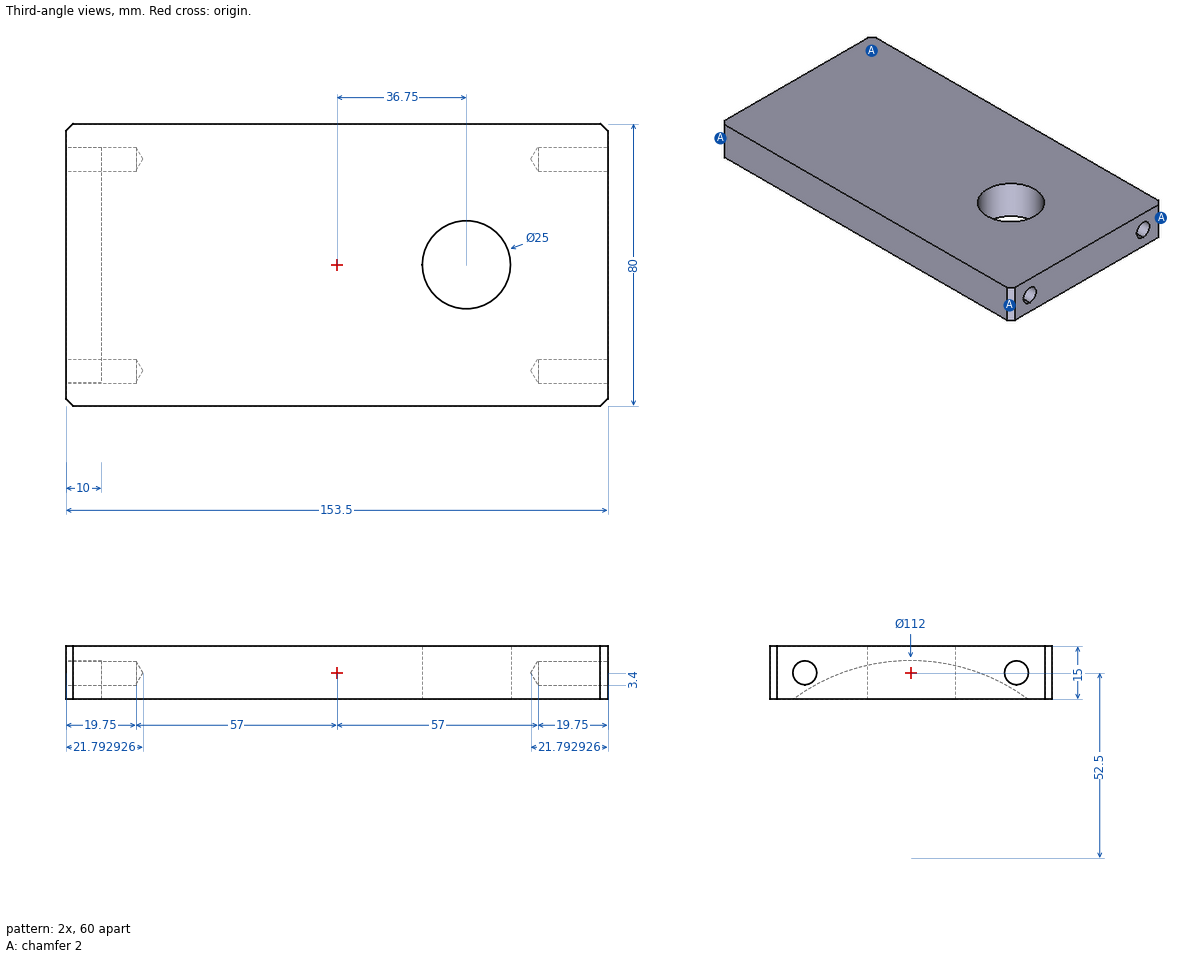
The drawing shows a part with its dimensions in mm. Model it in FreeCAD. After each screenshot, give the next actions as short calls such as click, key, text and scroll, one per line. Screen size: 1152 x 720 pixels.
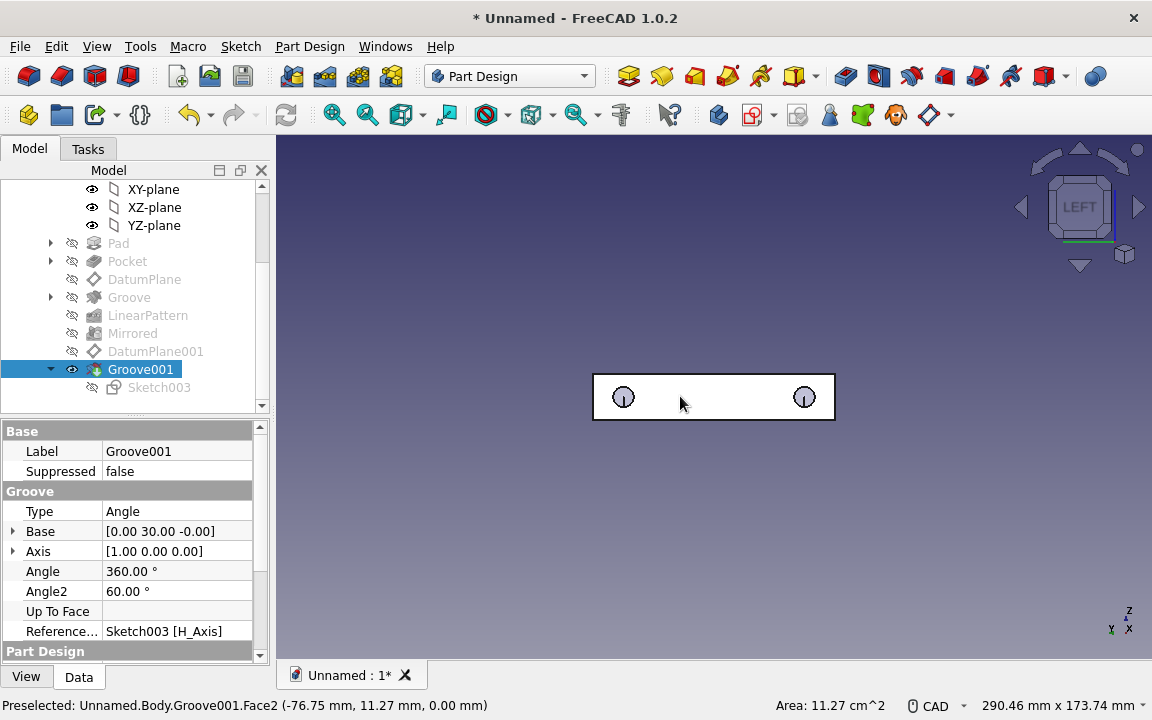
click(752, 116)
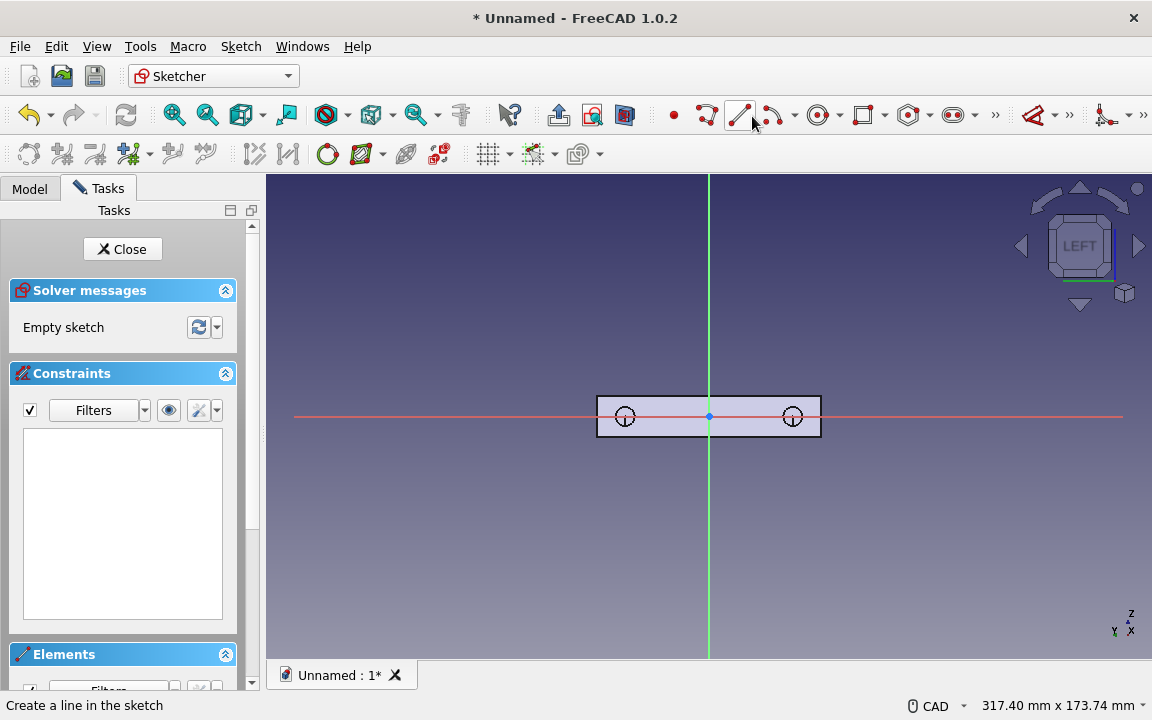
scroll(501, 202, down, 2)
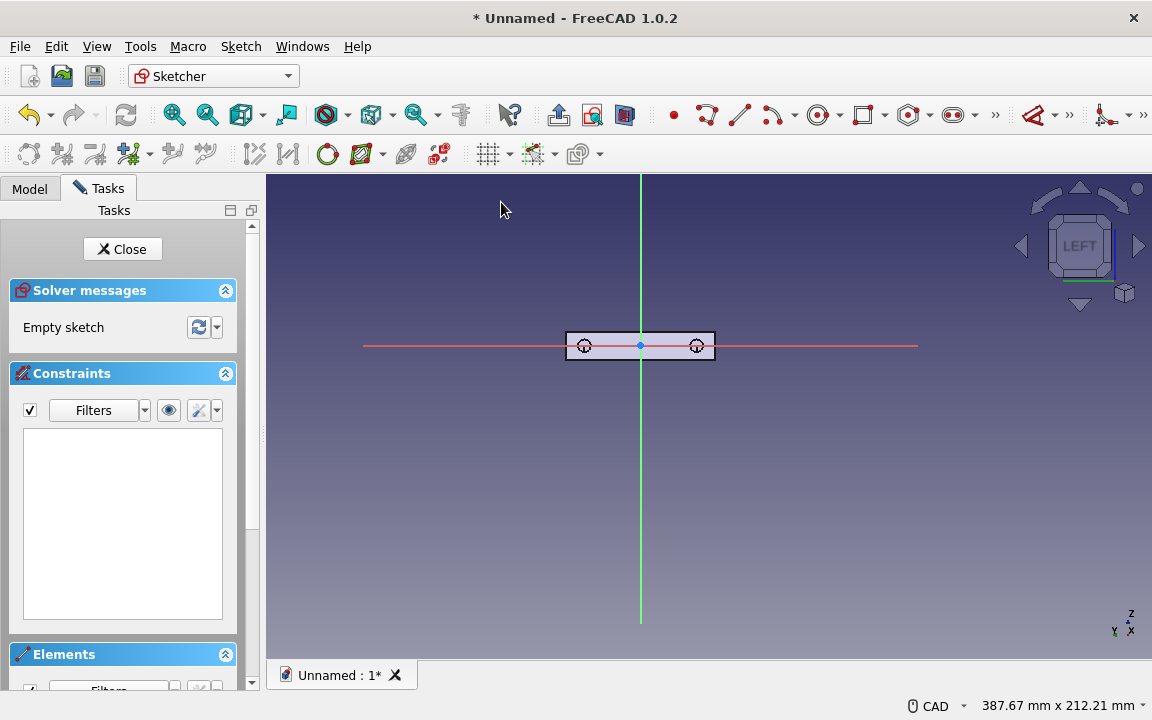
scroll(641, 500, up, 2)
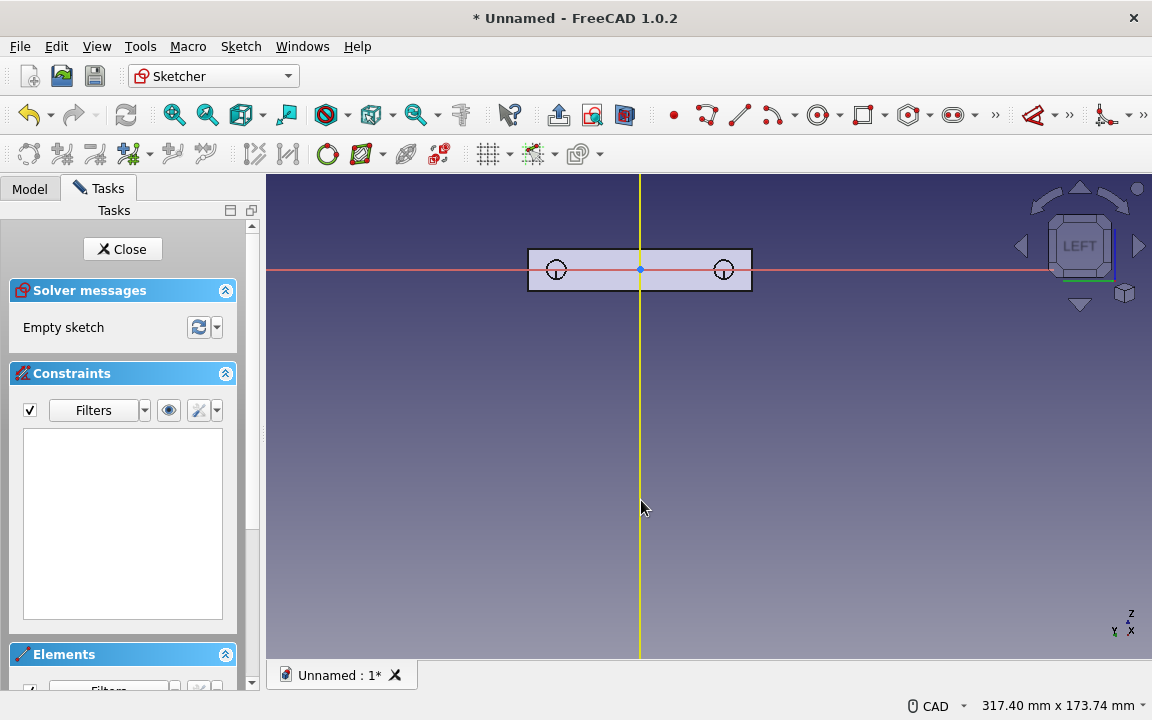
click(818, 116)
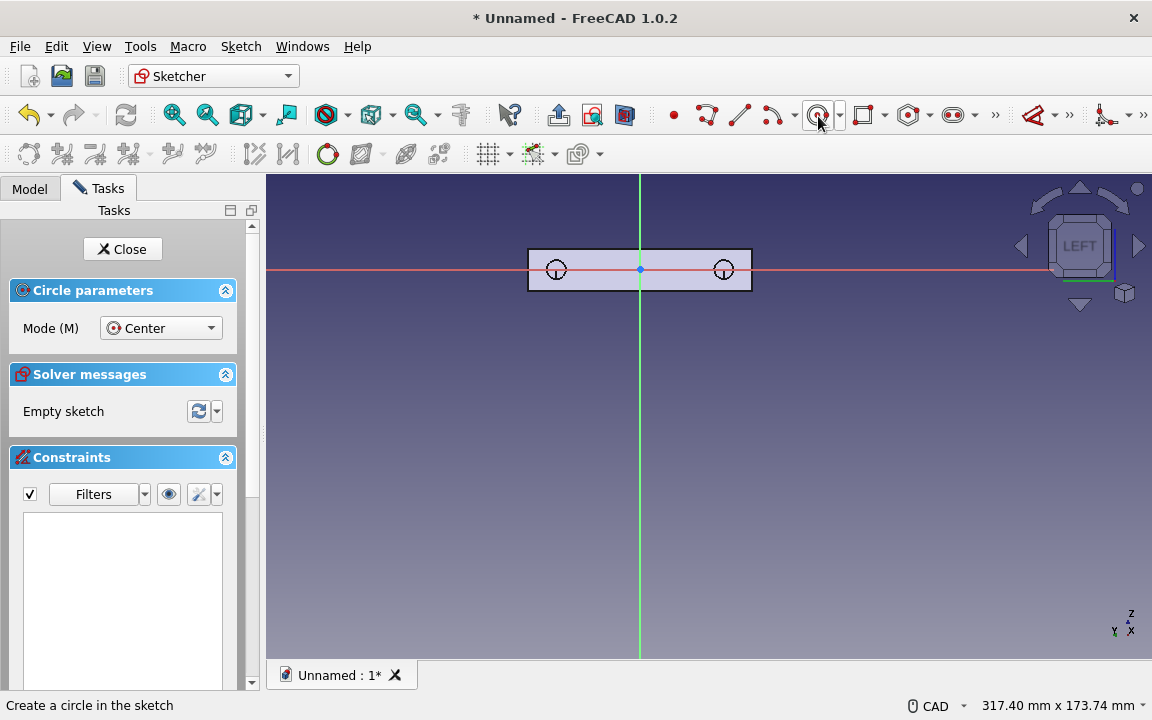
click(640, 416)
move(751, 306)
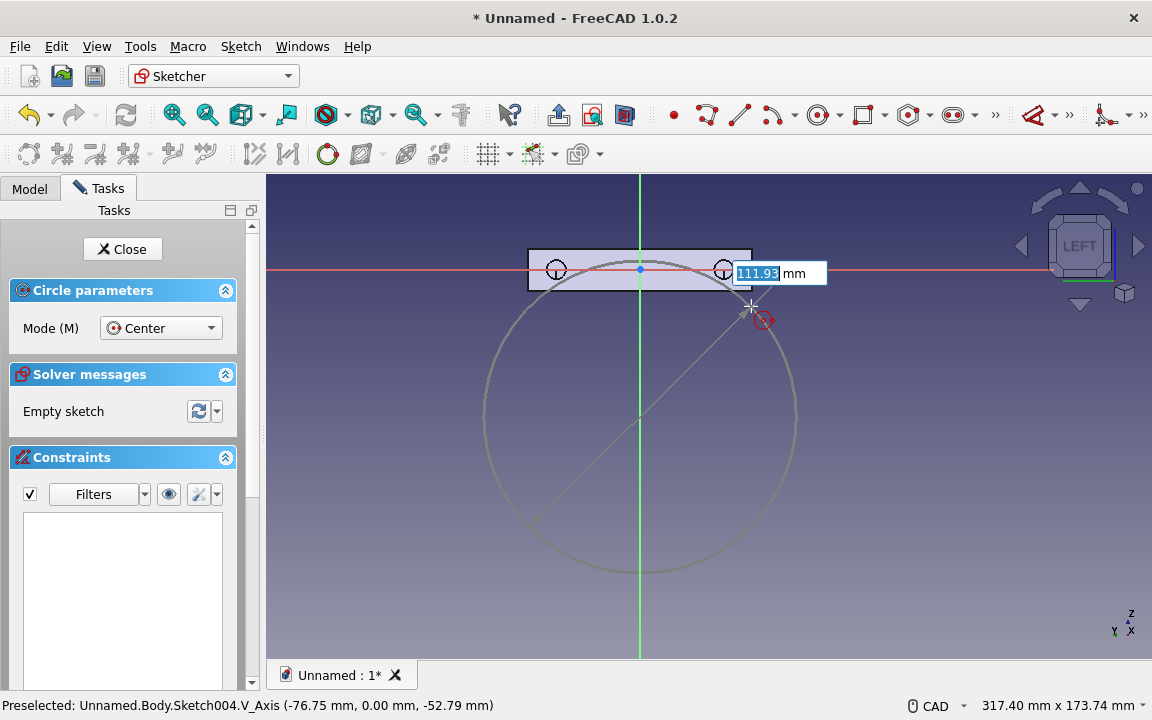
text(112)
key(Return)
key(Escape)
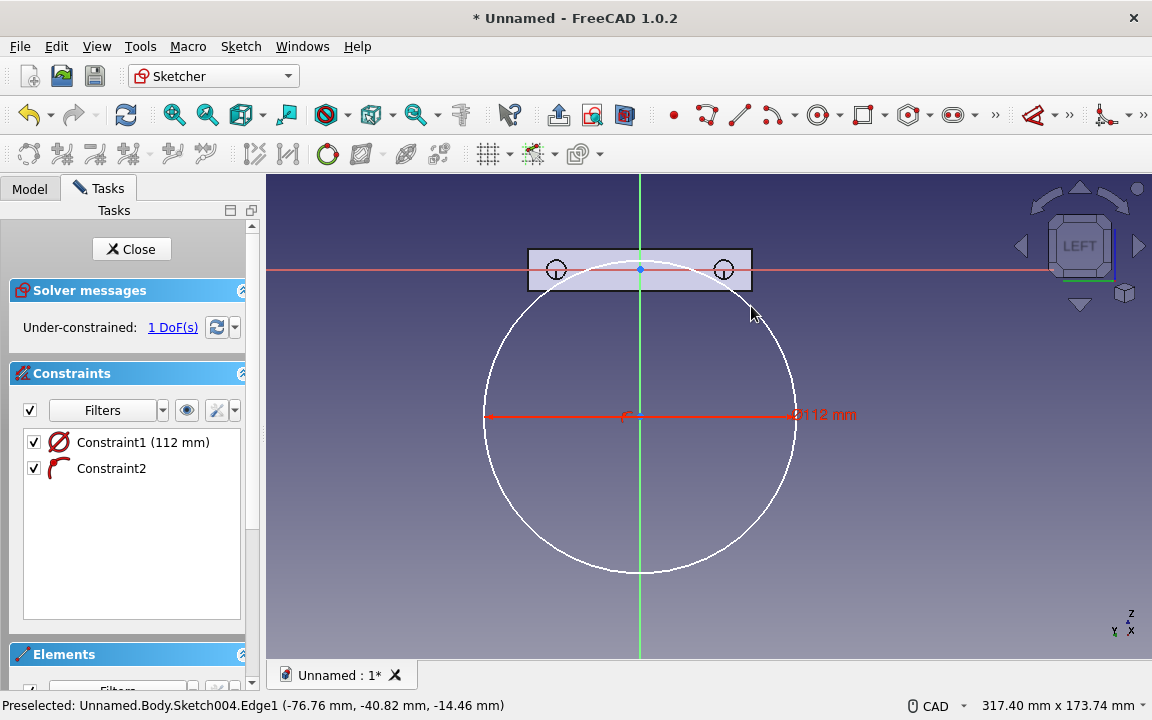
click(1032, 116)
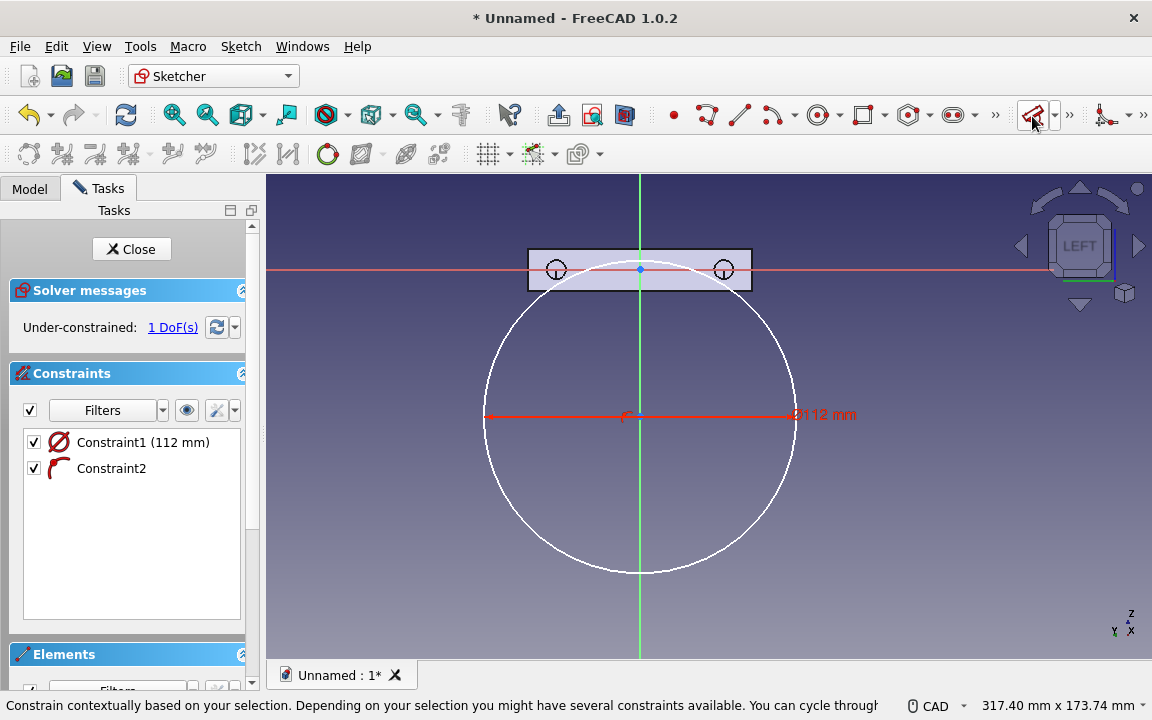
click(640, 417)
click(674, 343)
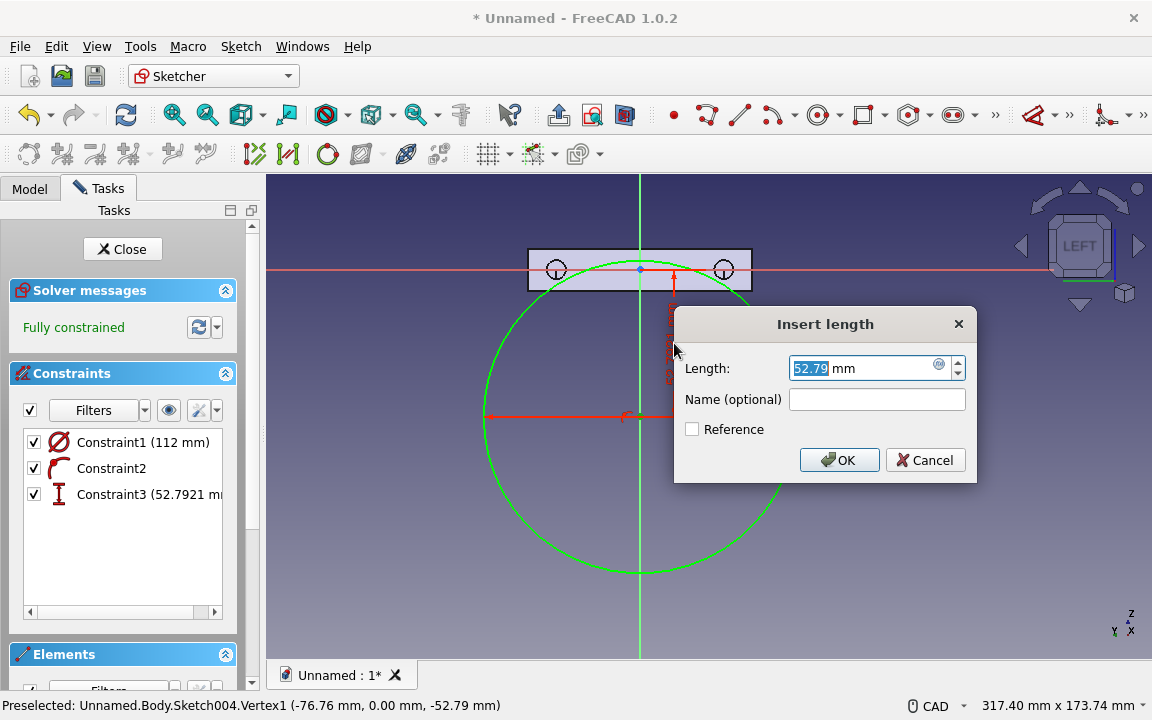
text(52.5)
key(Return)
key(Escape)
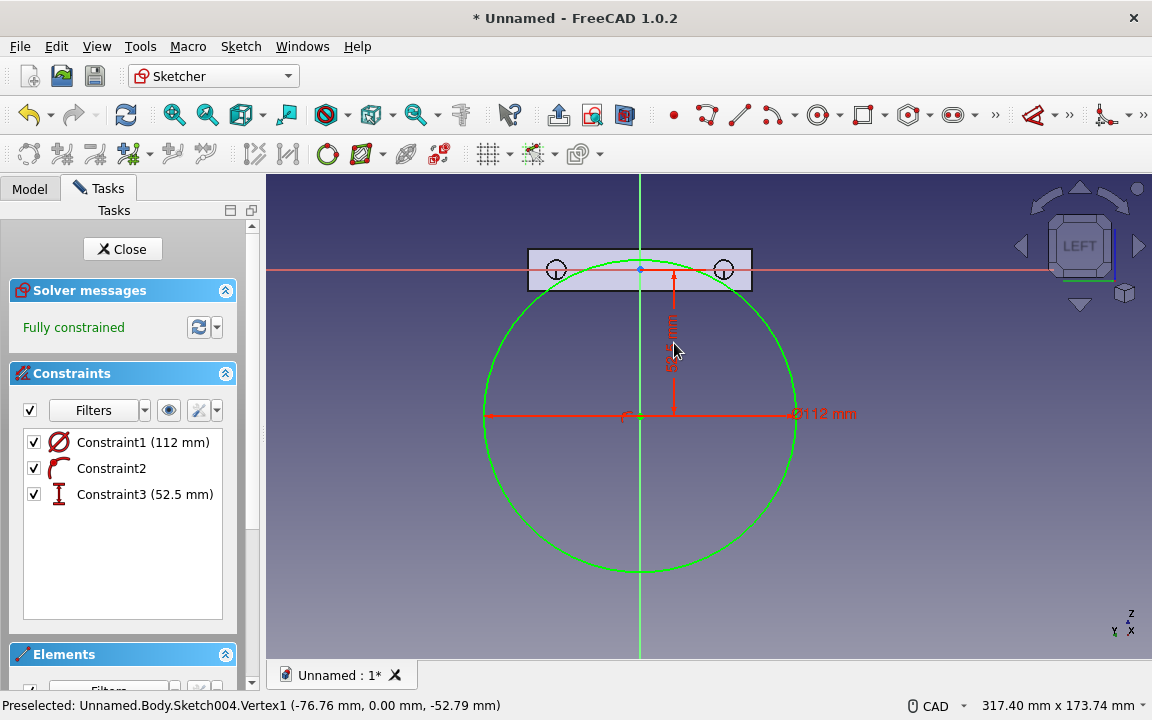
click(123, 249)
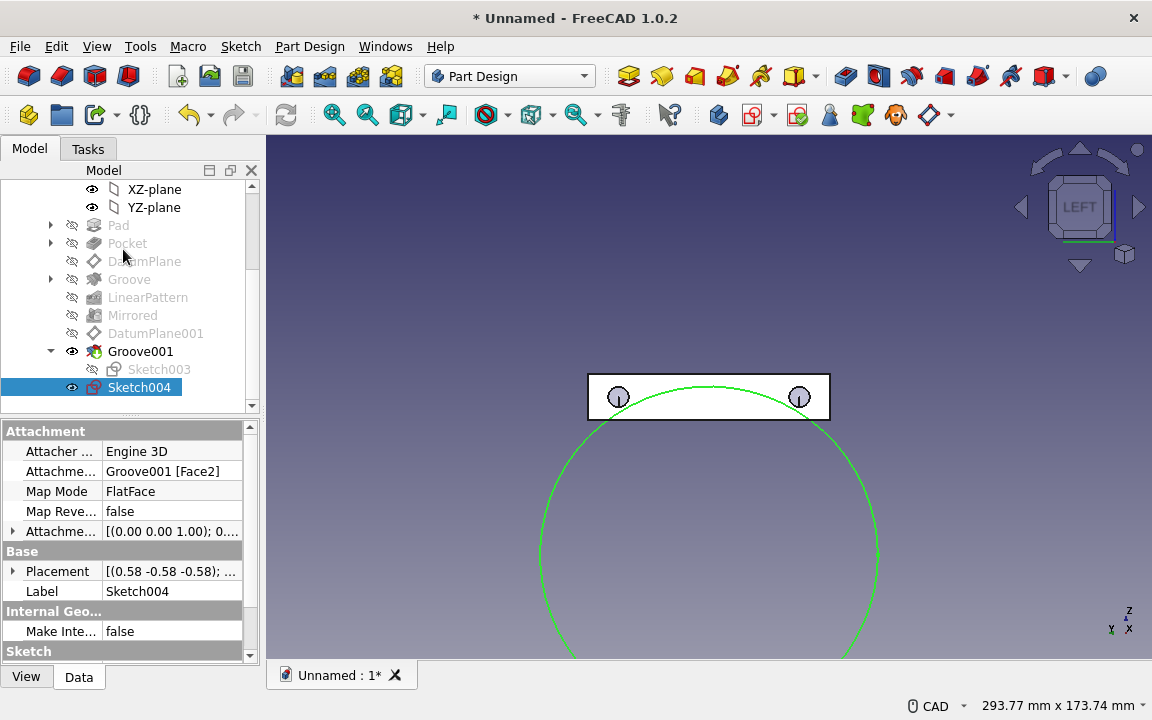
click(846, 76)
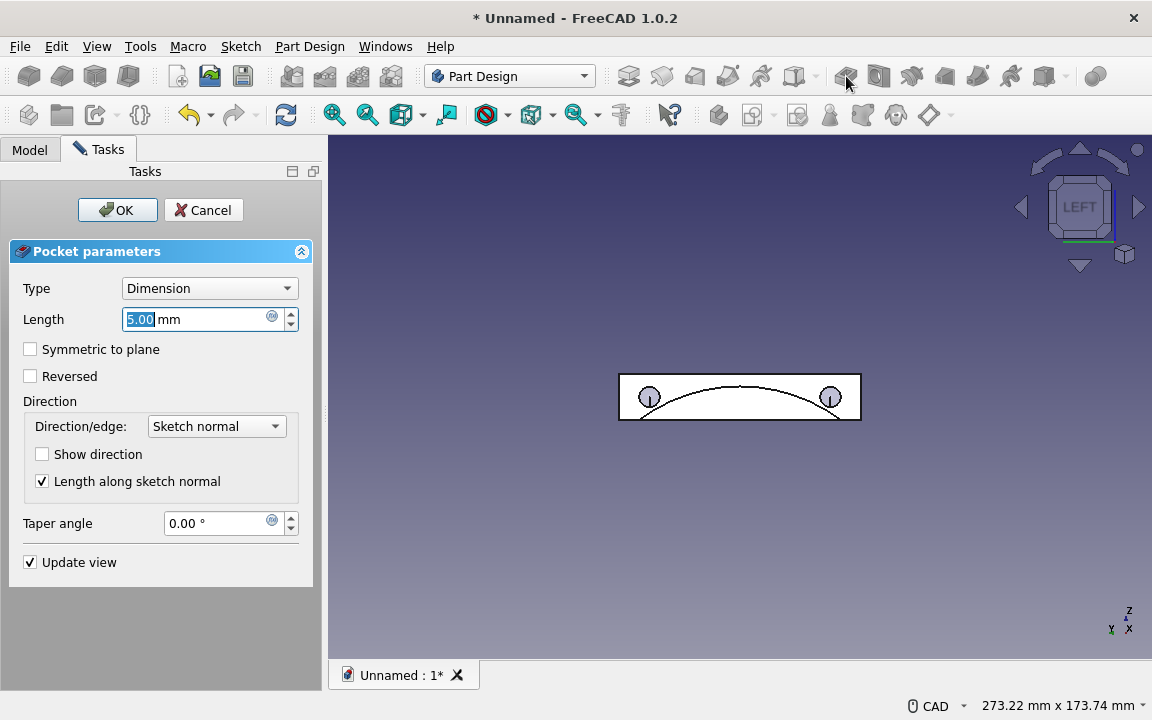
text(10)
key(Tab)